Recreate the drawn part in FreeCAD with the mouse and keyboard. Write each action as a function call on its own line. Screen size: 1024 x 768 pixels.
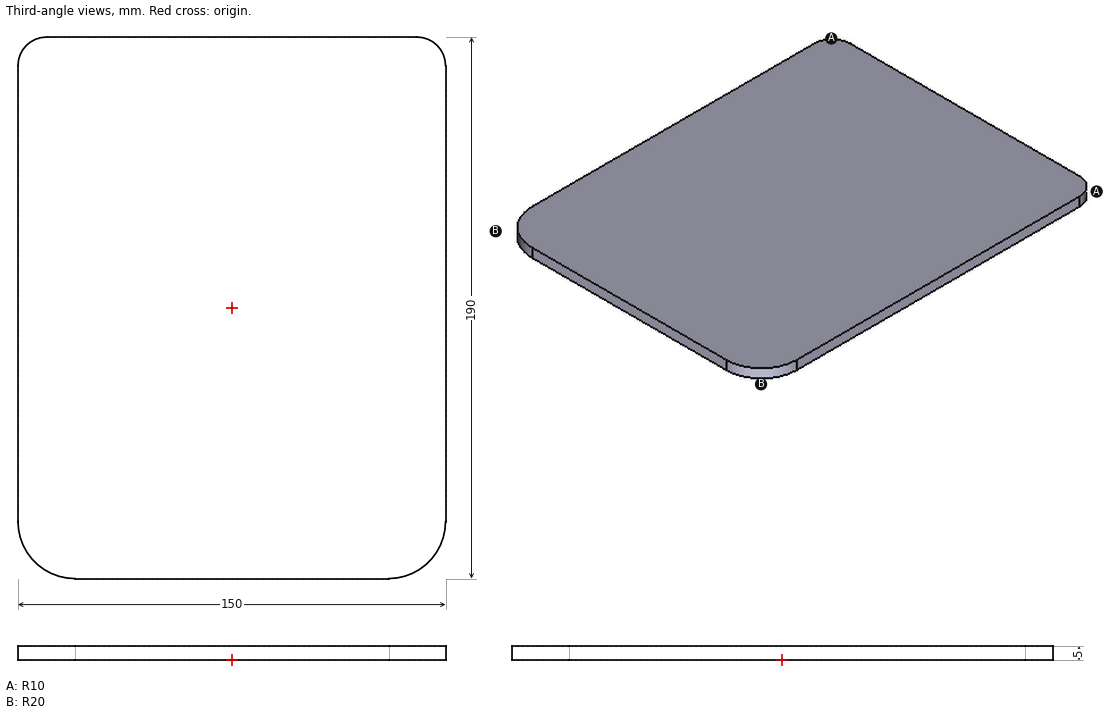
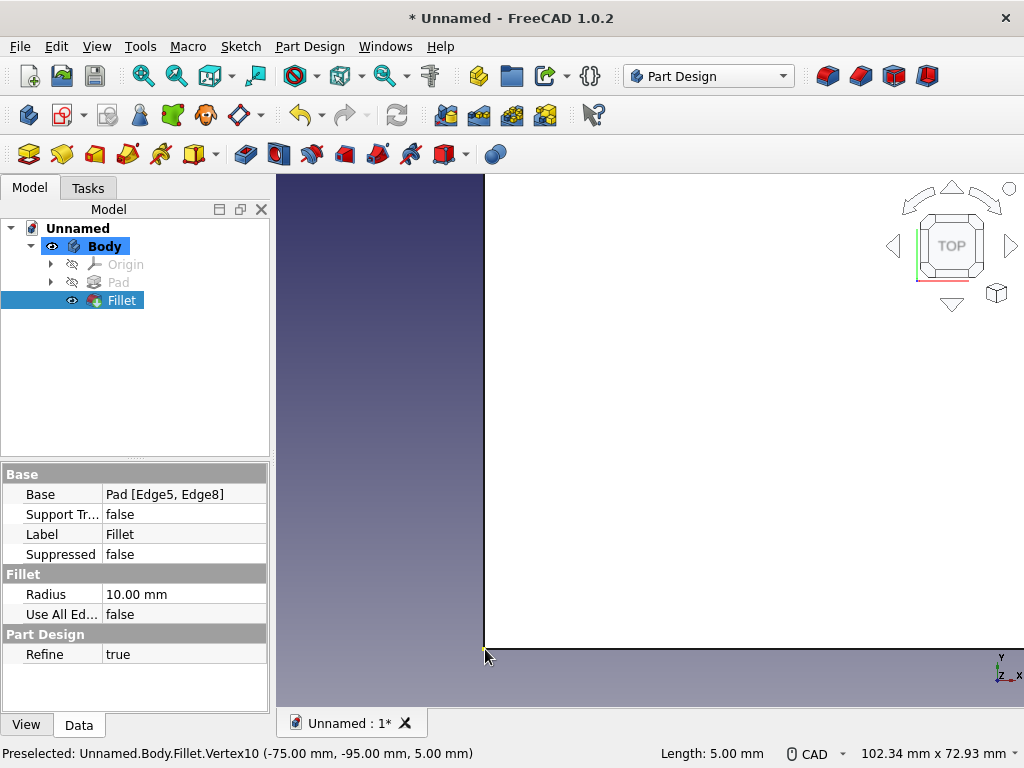
click(144, 76)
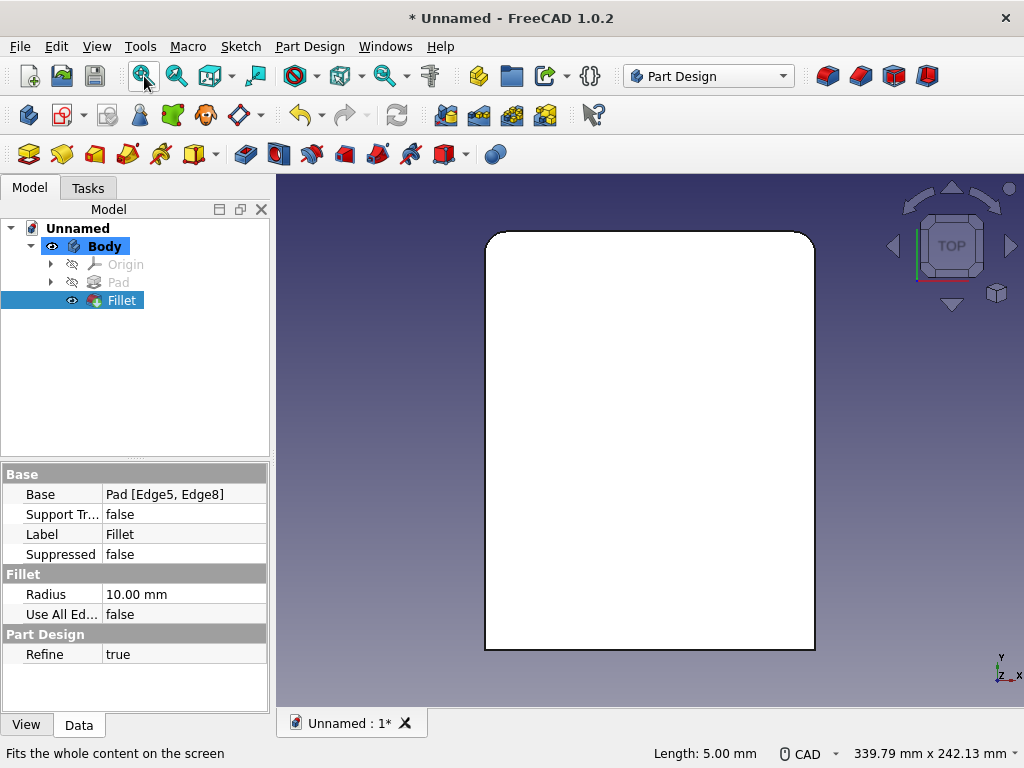
key(1)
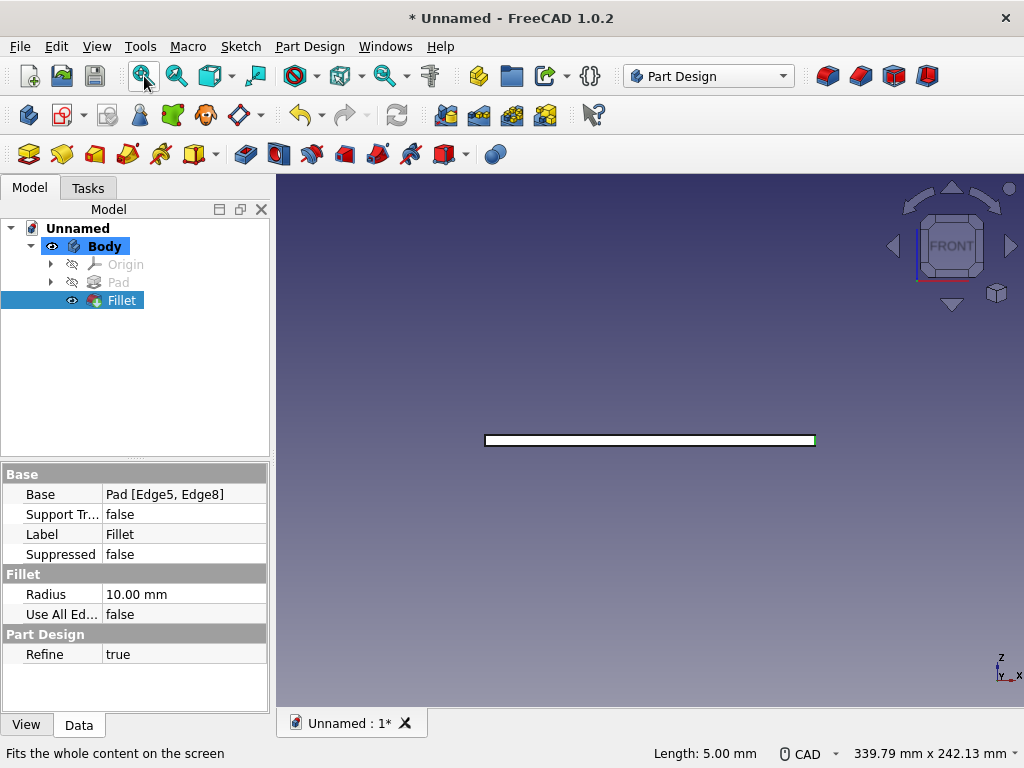
click(144, 76)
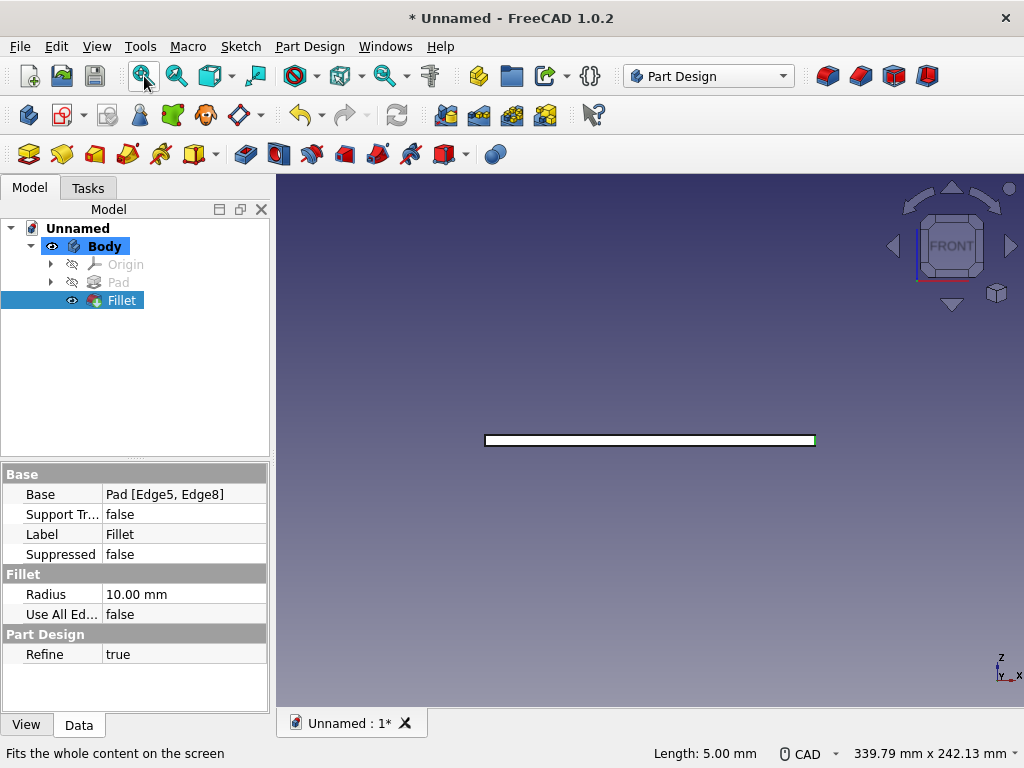
scroll(485, 440, up, 7)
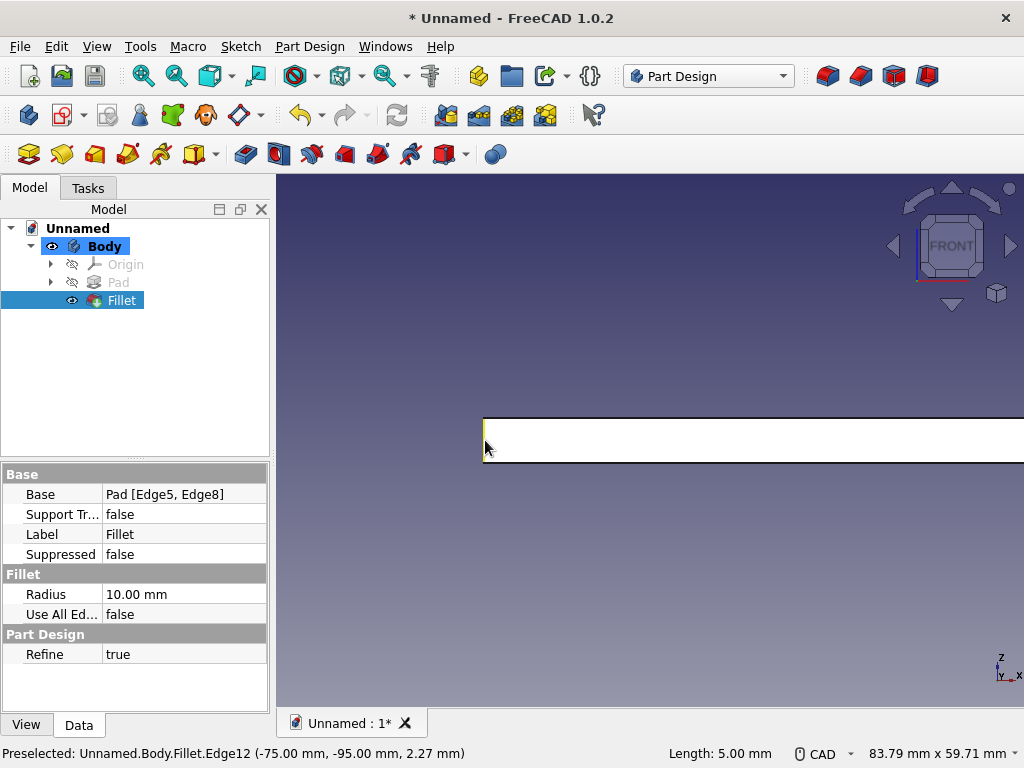
click(484, 440, ctrl)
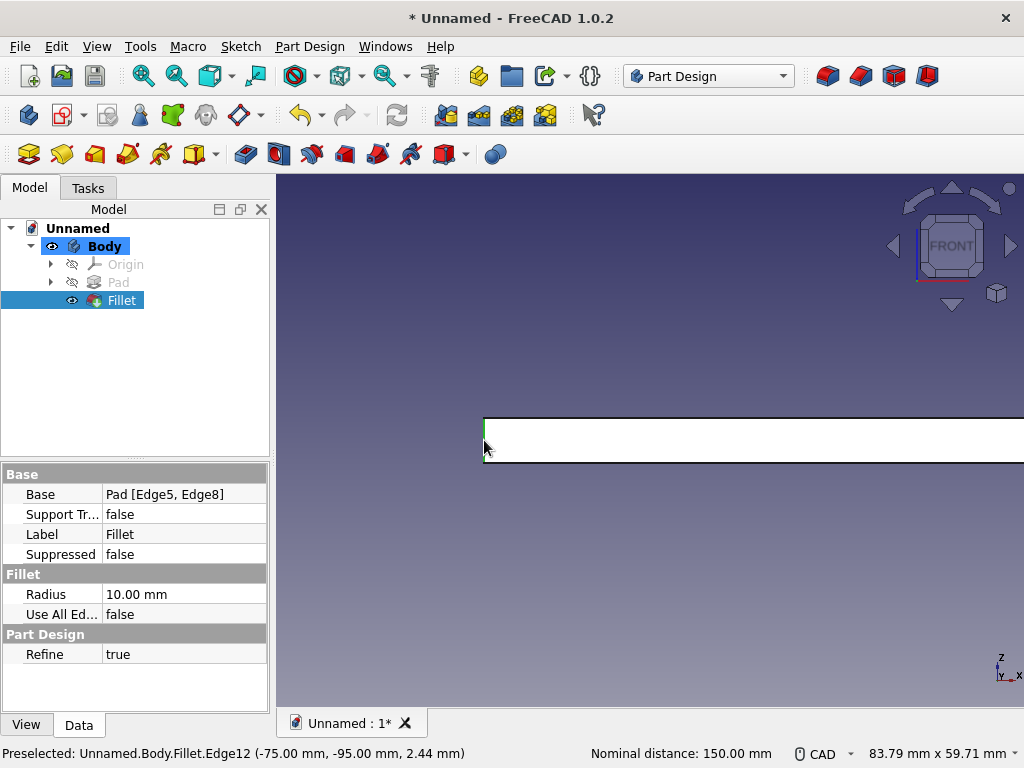
click(828, 76)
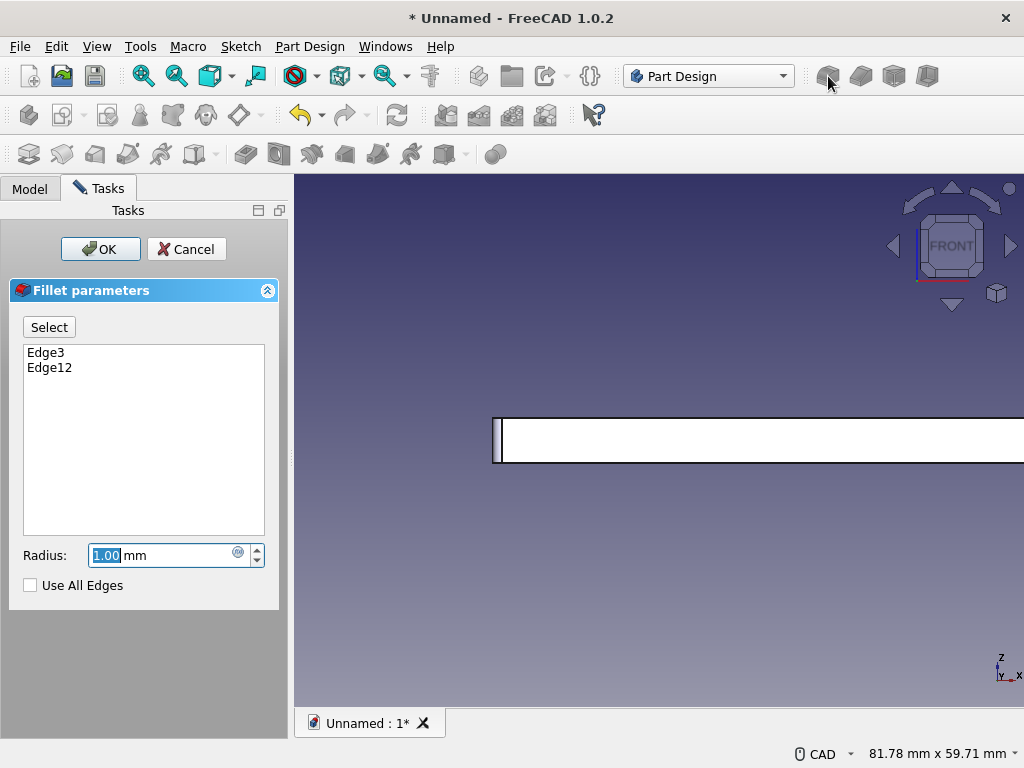
text(20)
key(Tab)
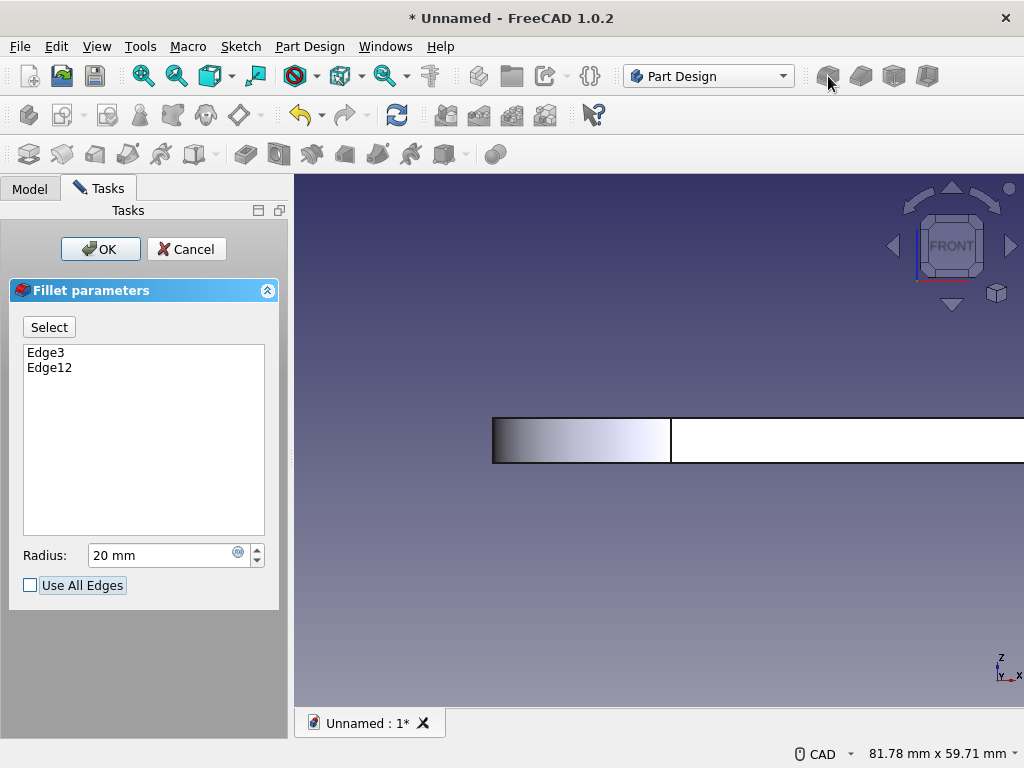
click(101, 249)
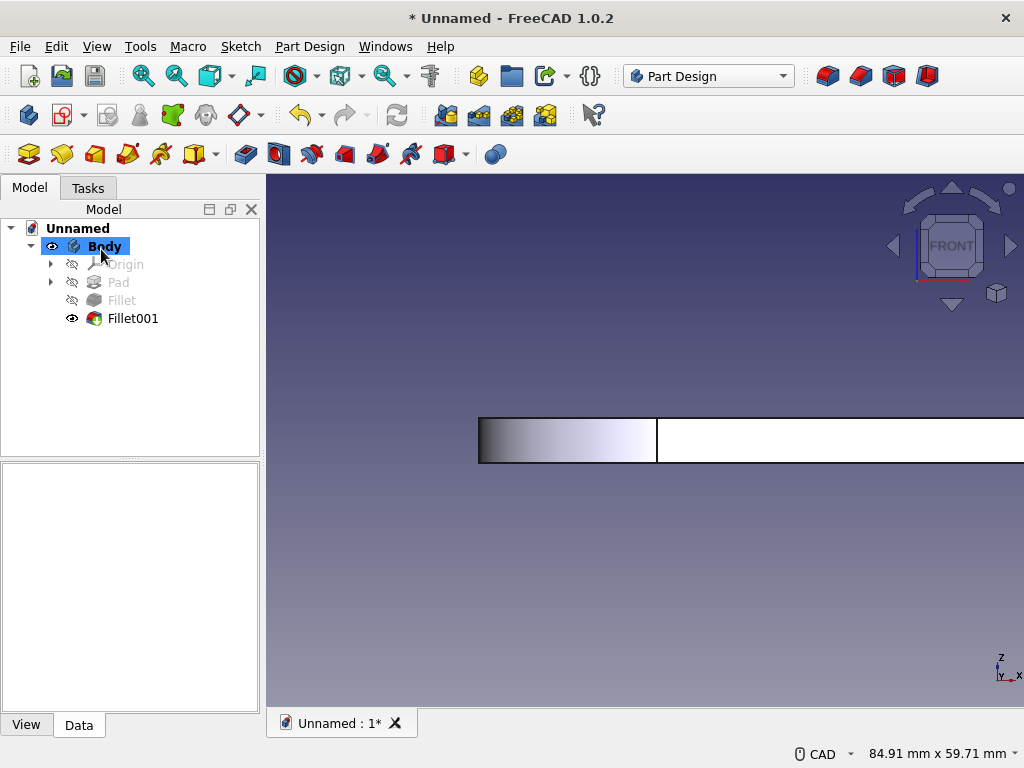
key(0)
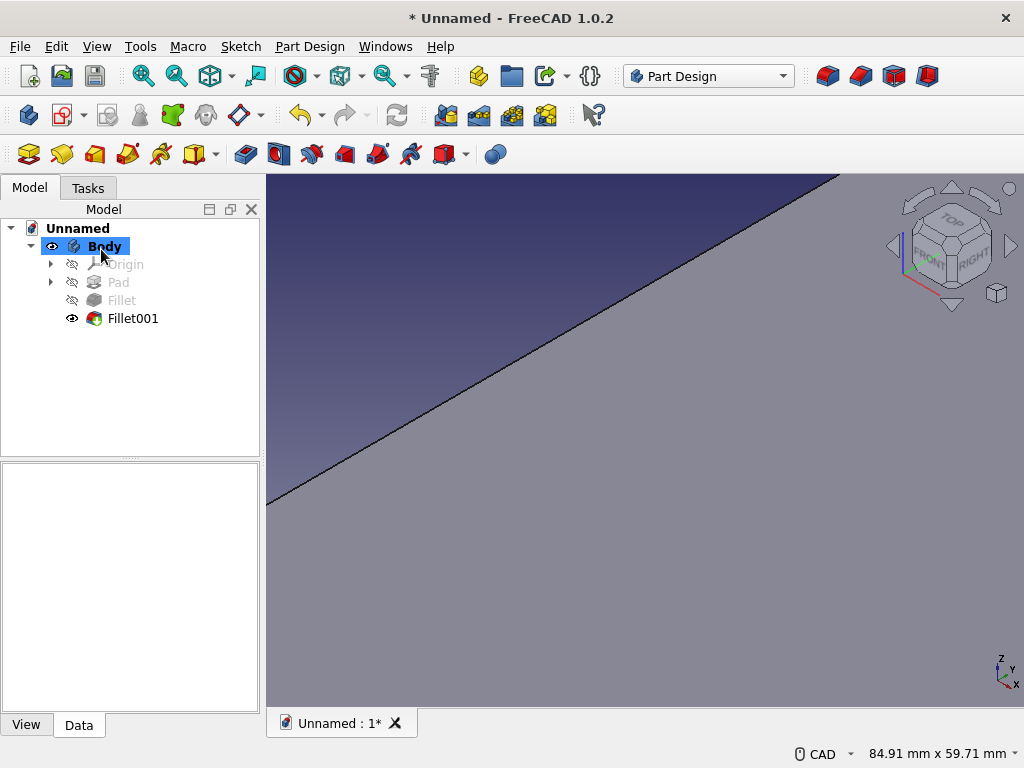
click(144, 76)